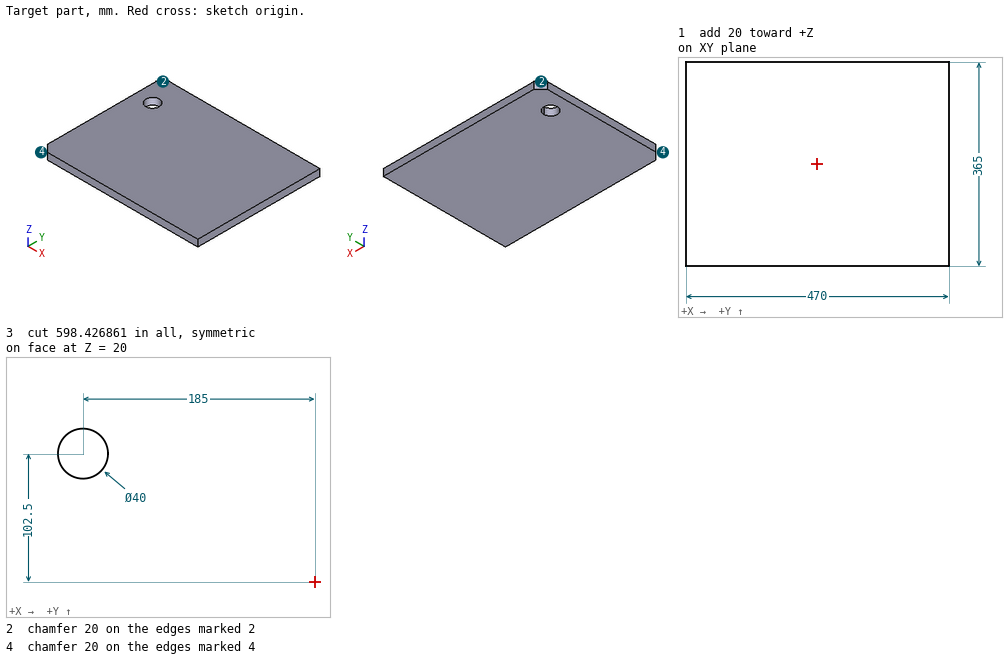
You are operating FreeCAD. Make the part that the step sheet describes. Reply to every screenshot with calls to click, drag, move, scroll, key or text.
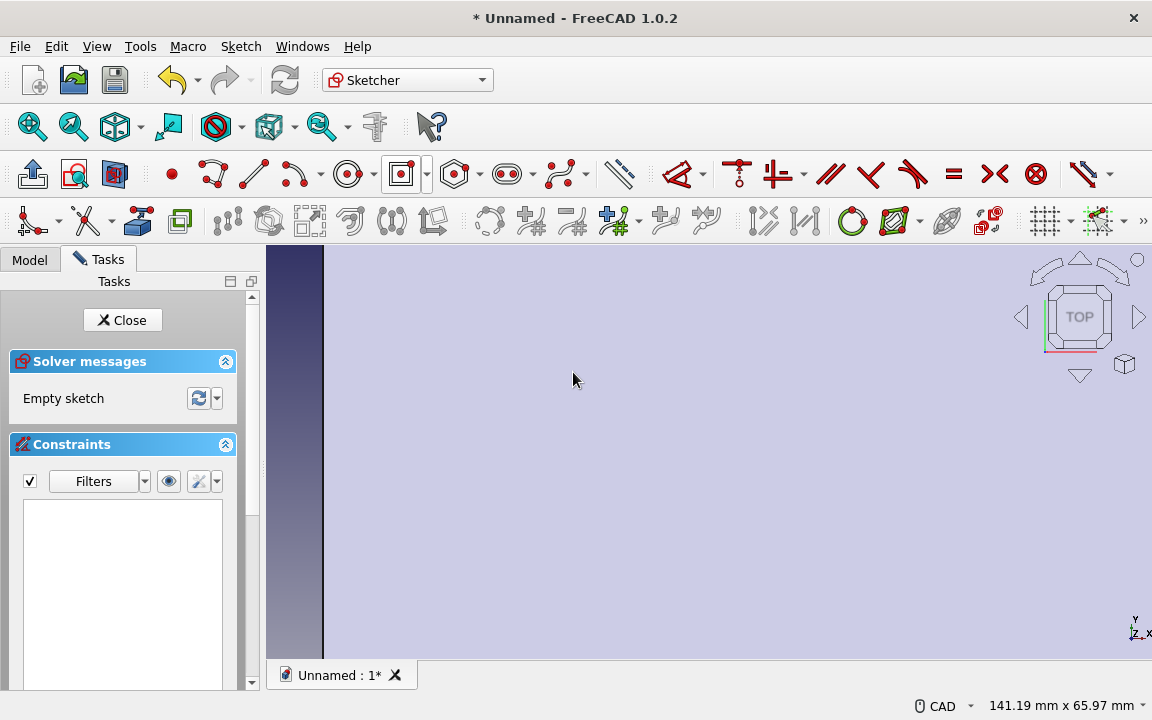
click(348, 174)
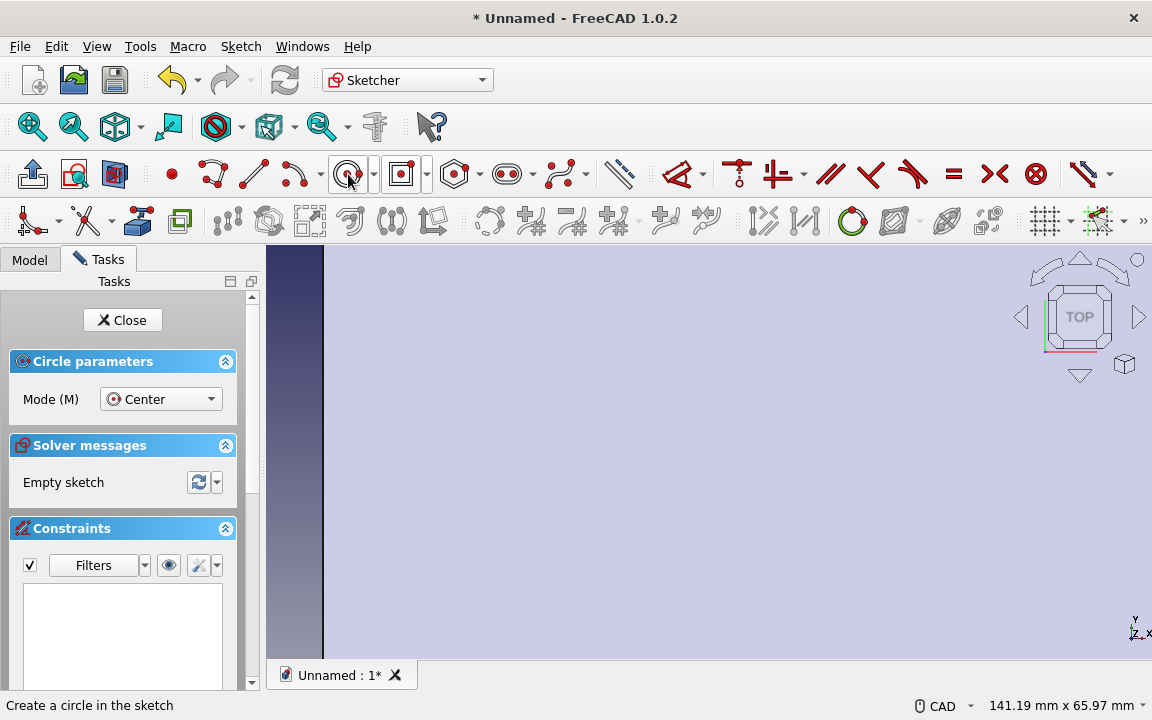
click(637, 448)
click(725, 360)
key(Escape)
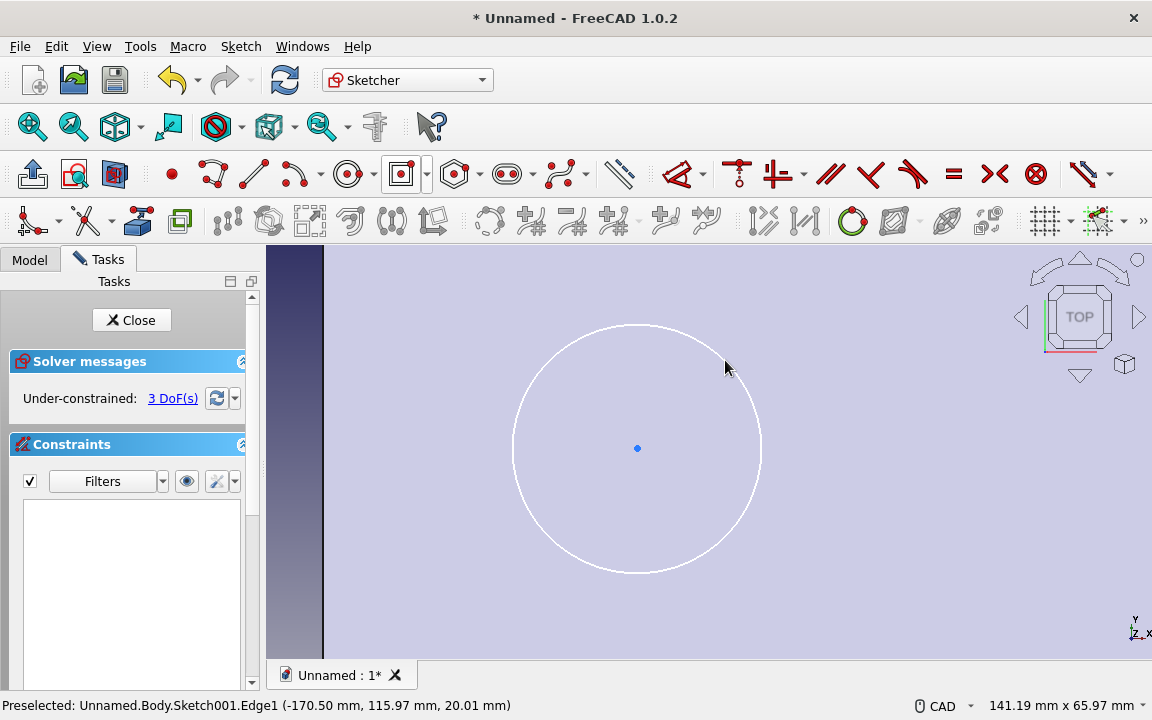
click(676, 174)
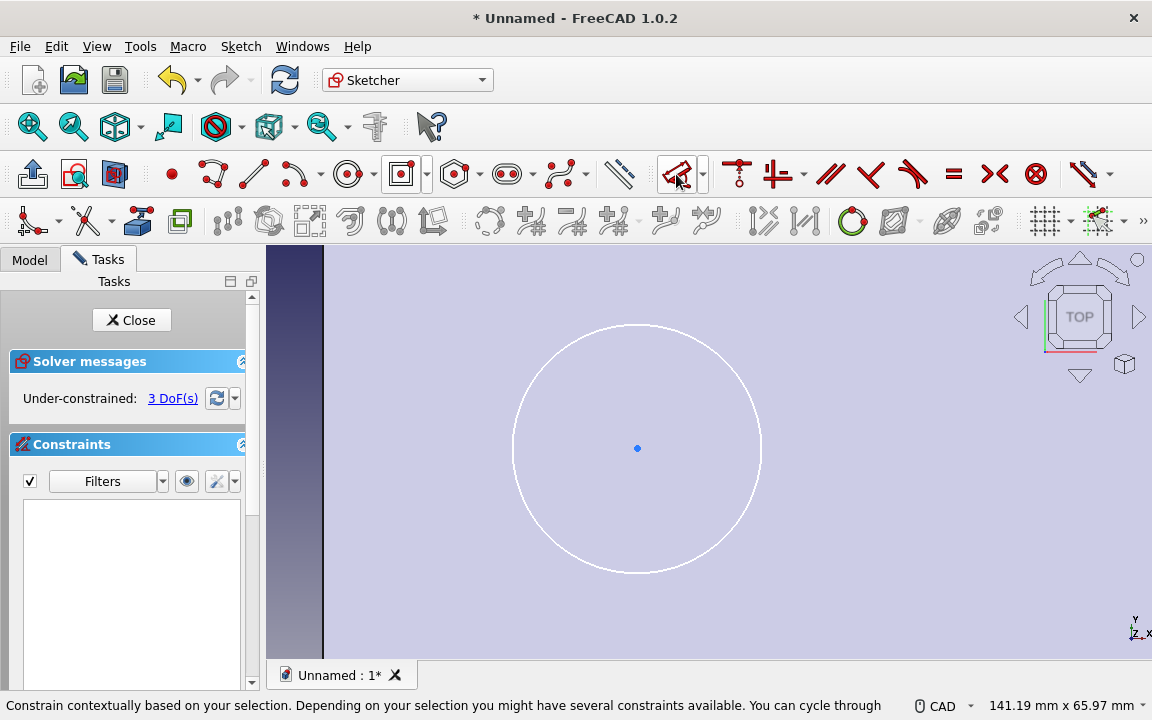
click(725, 361)
click(748, 338)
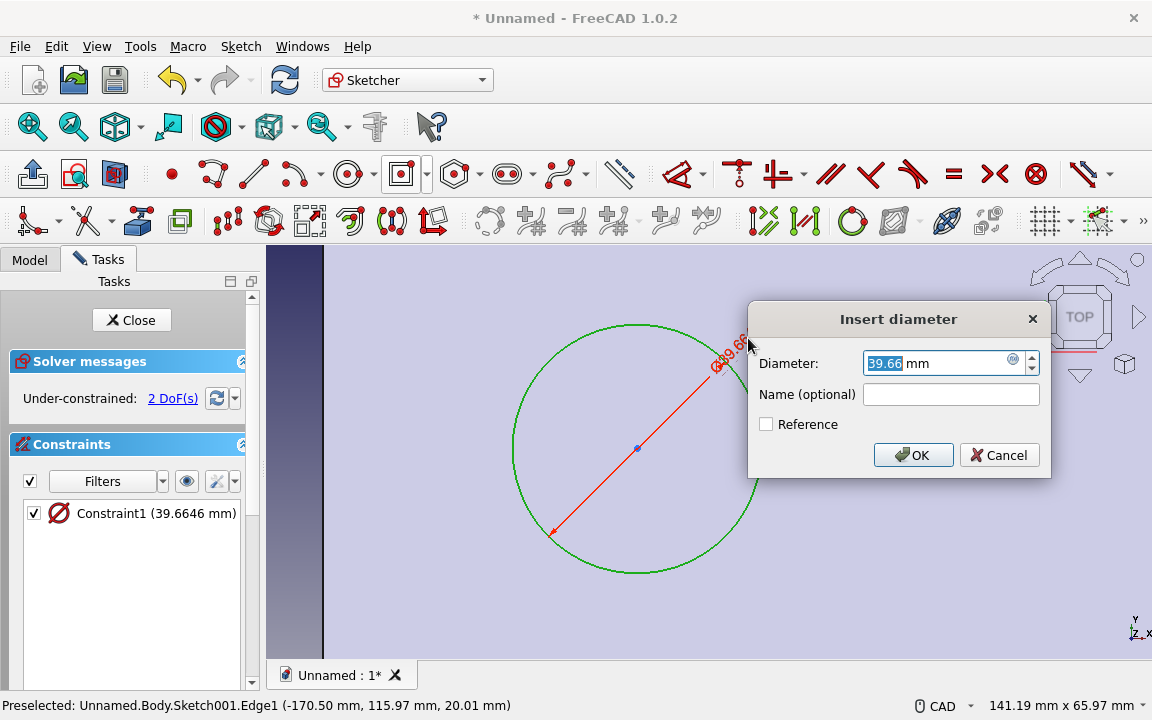
text(40)
key(Return)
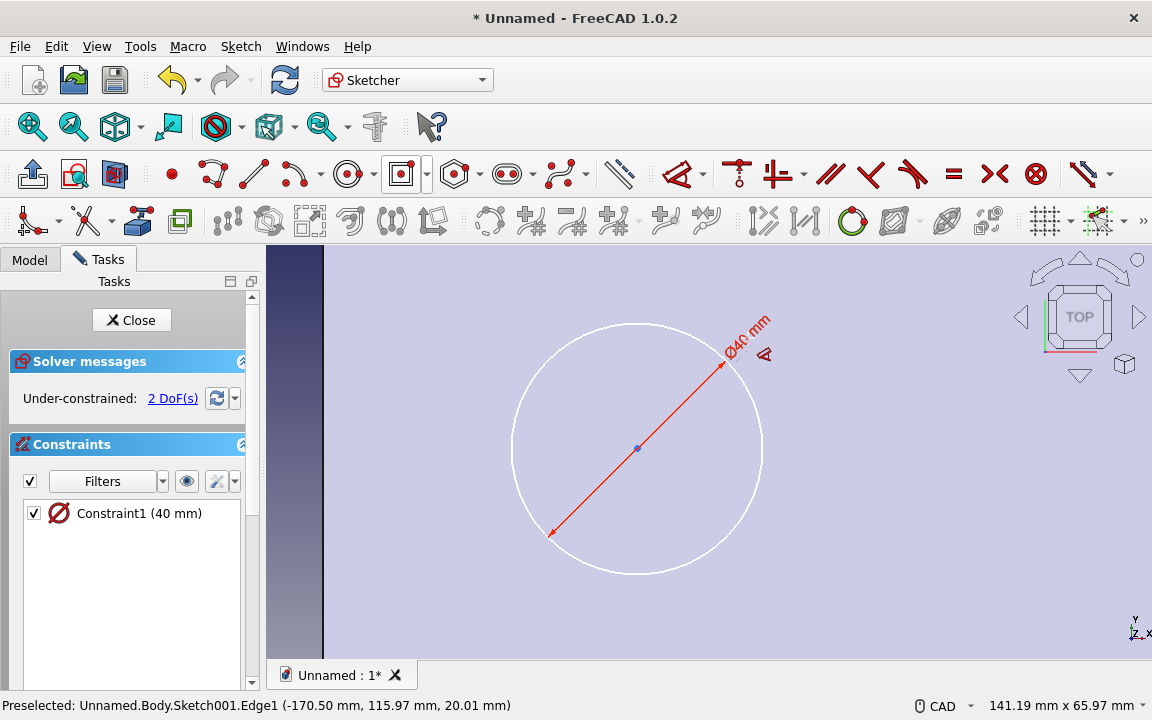
click(637, 449)
click(812, 415)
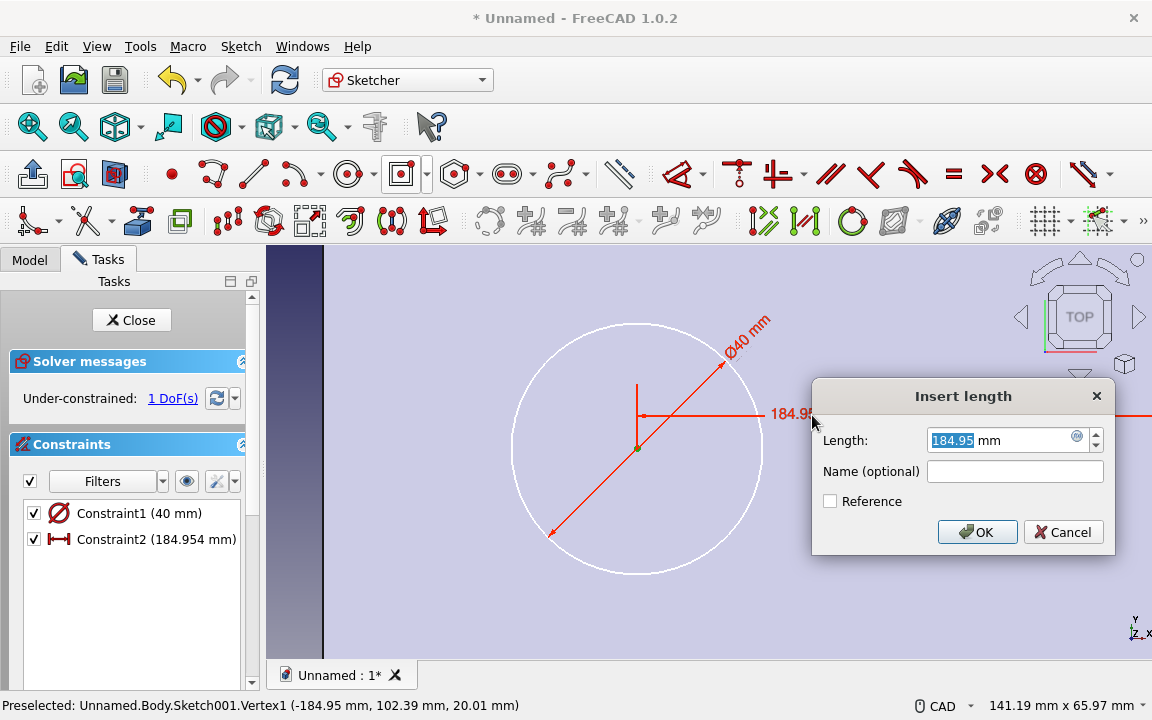
text(185)
key(Return)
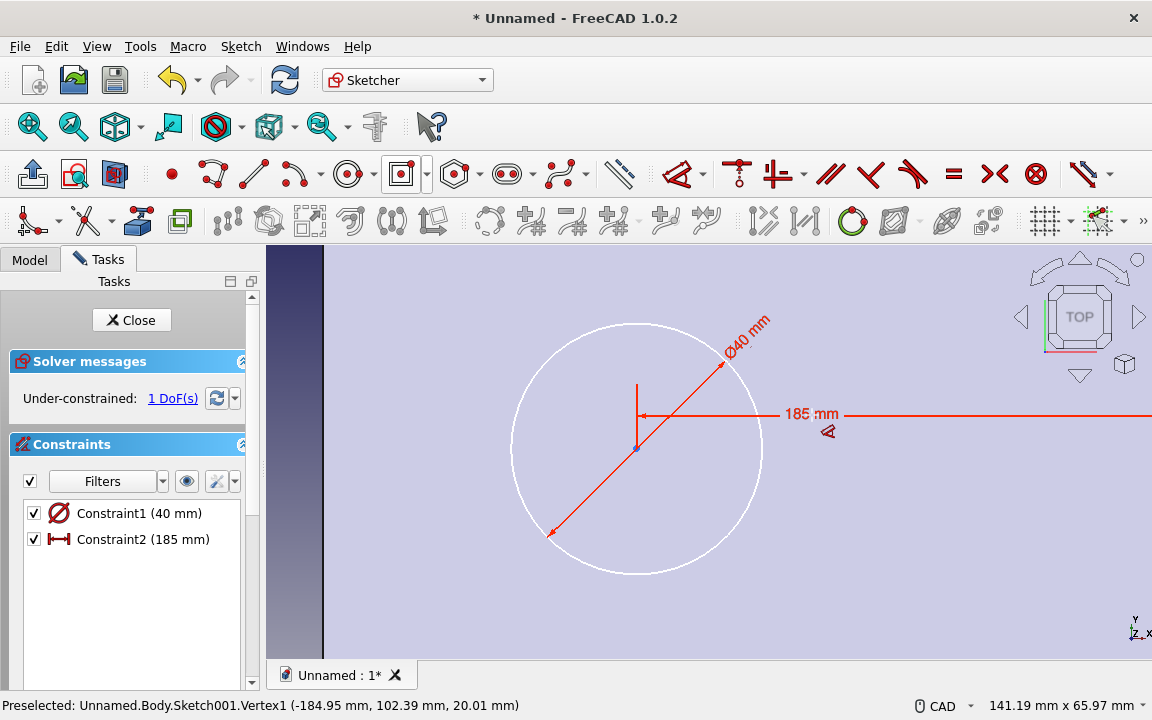
click(637, 449)
click(603, 540)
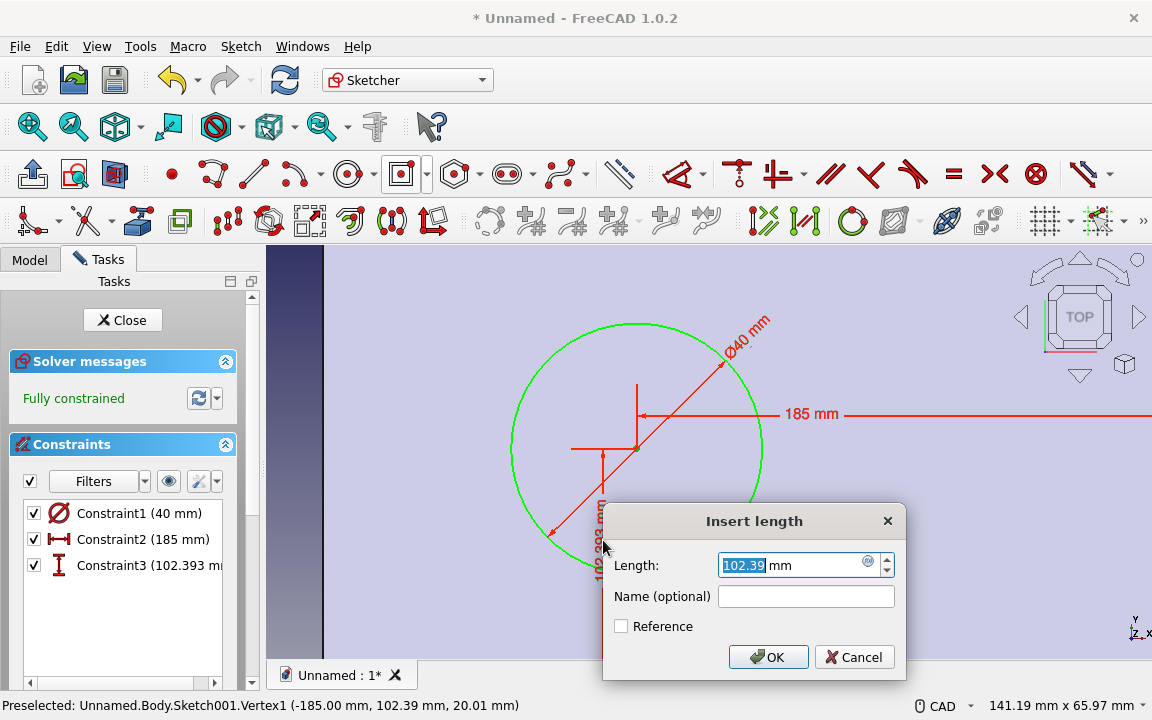
text(102.5)
key(Return)
key(Escape)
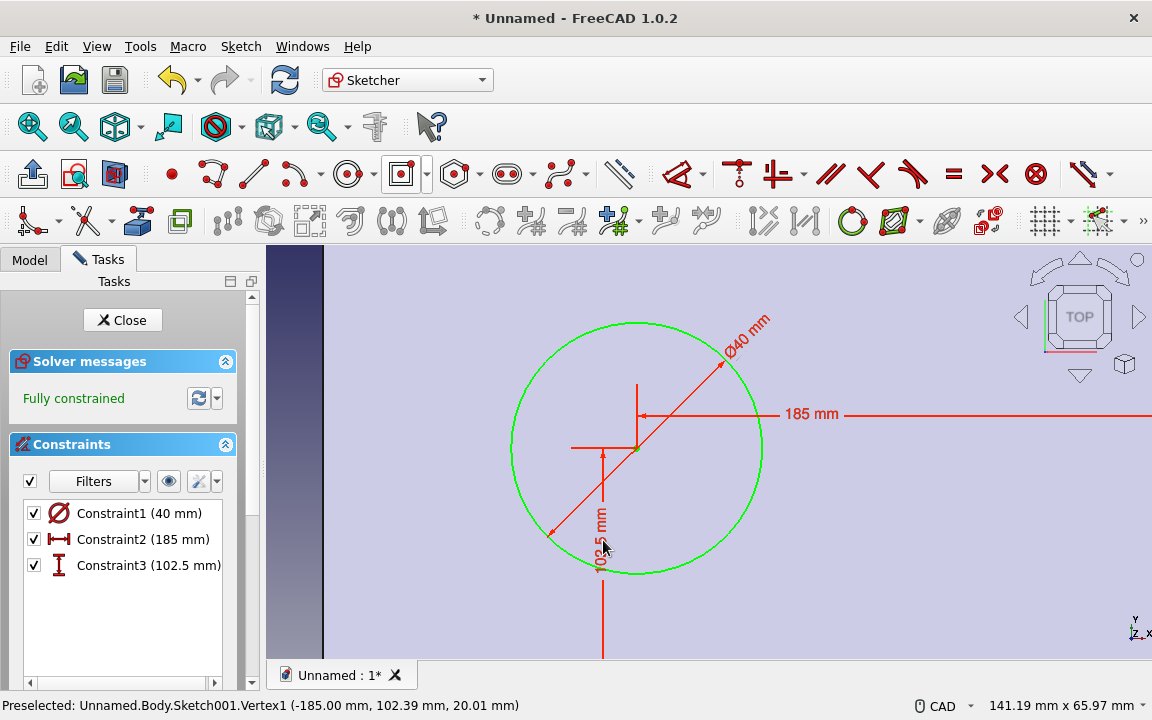
click(123, 320)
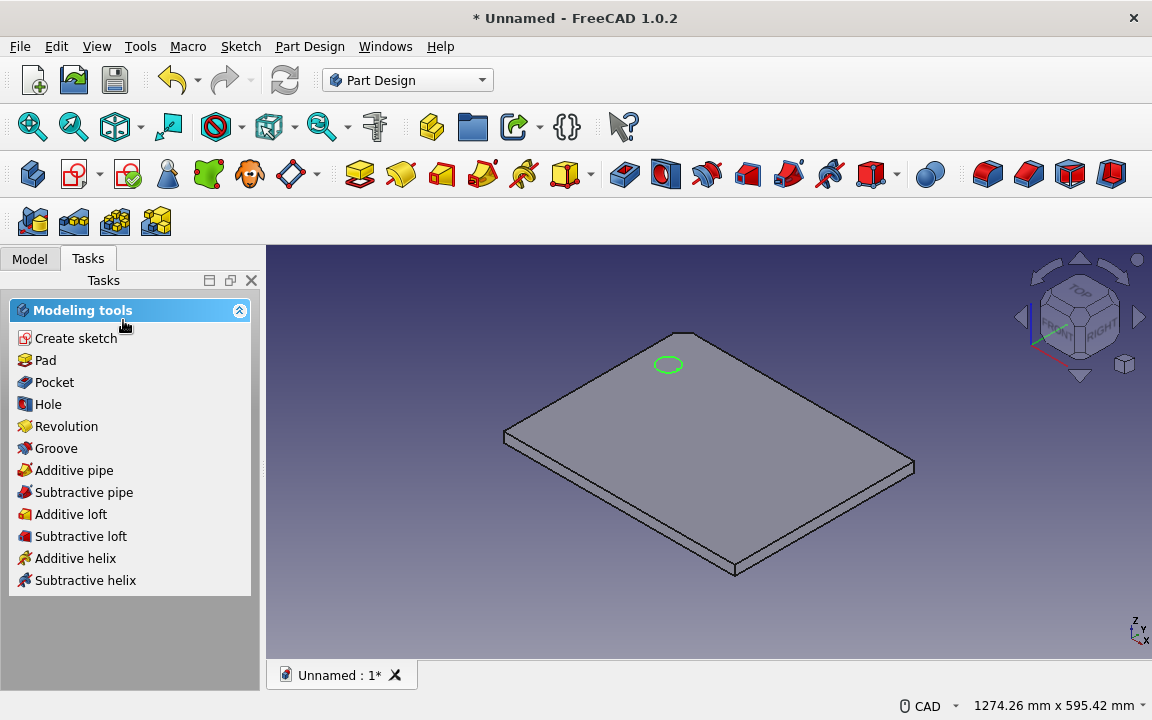
click(625, 174)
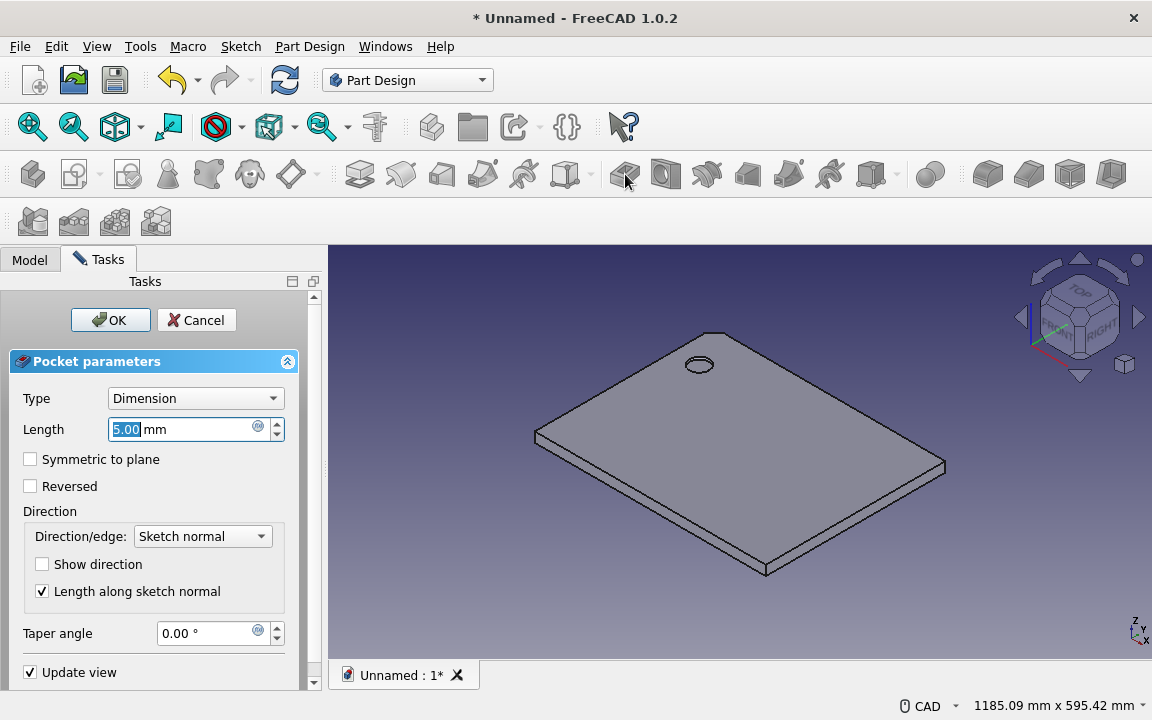
text(598.426861)
key(Tab)